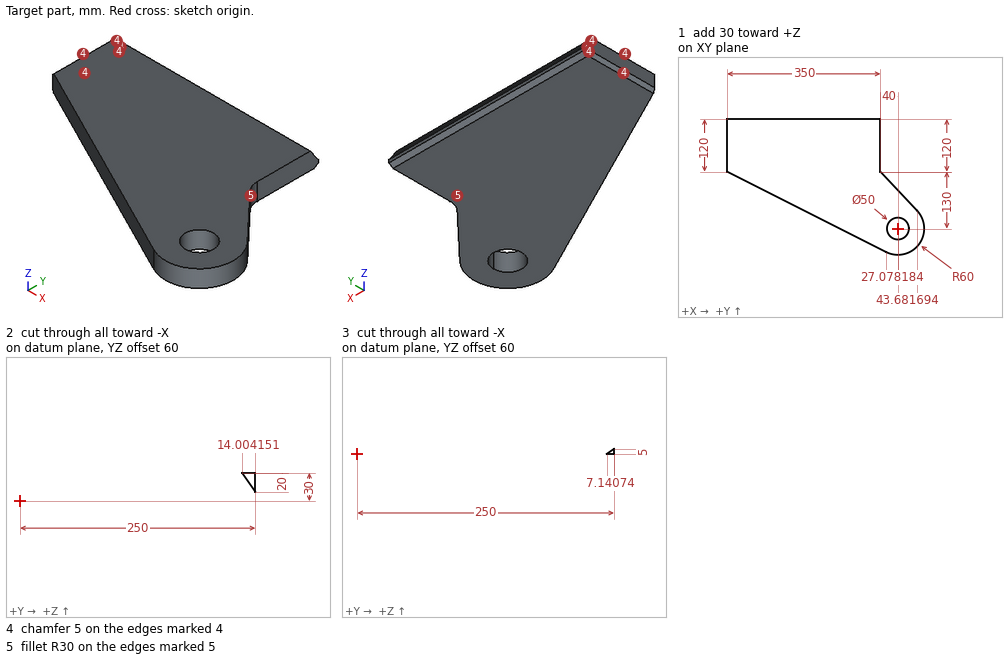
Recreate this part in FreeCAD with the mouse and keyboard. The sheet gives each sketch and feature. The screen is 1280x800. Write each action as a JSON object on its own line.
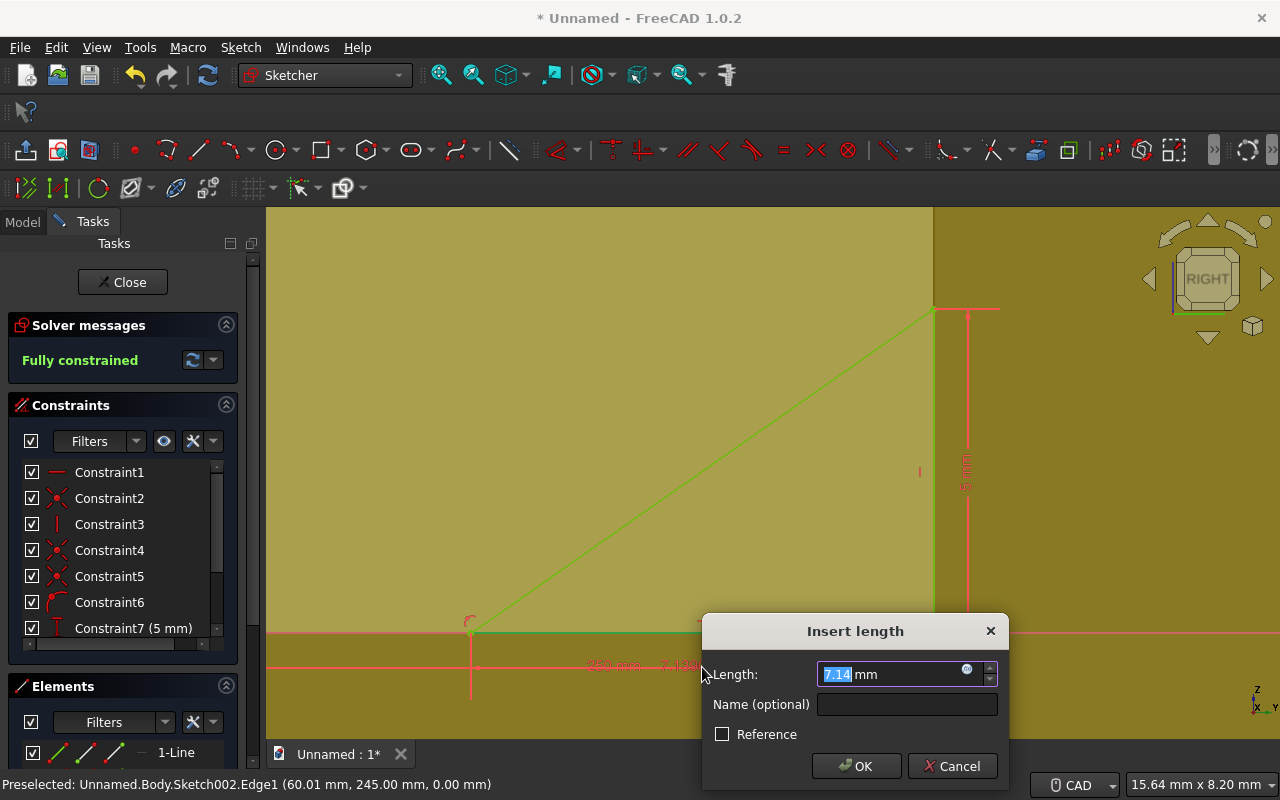
{"action": "type", "text": "7.14074"}
{"action": "key", "text": "Return"}
{"action": "key", "text": "Escape"}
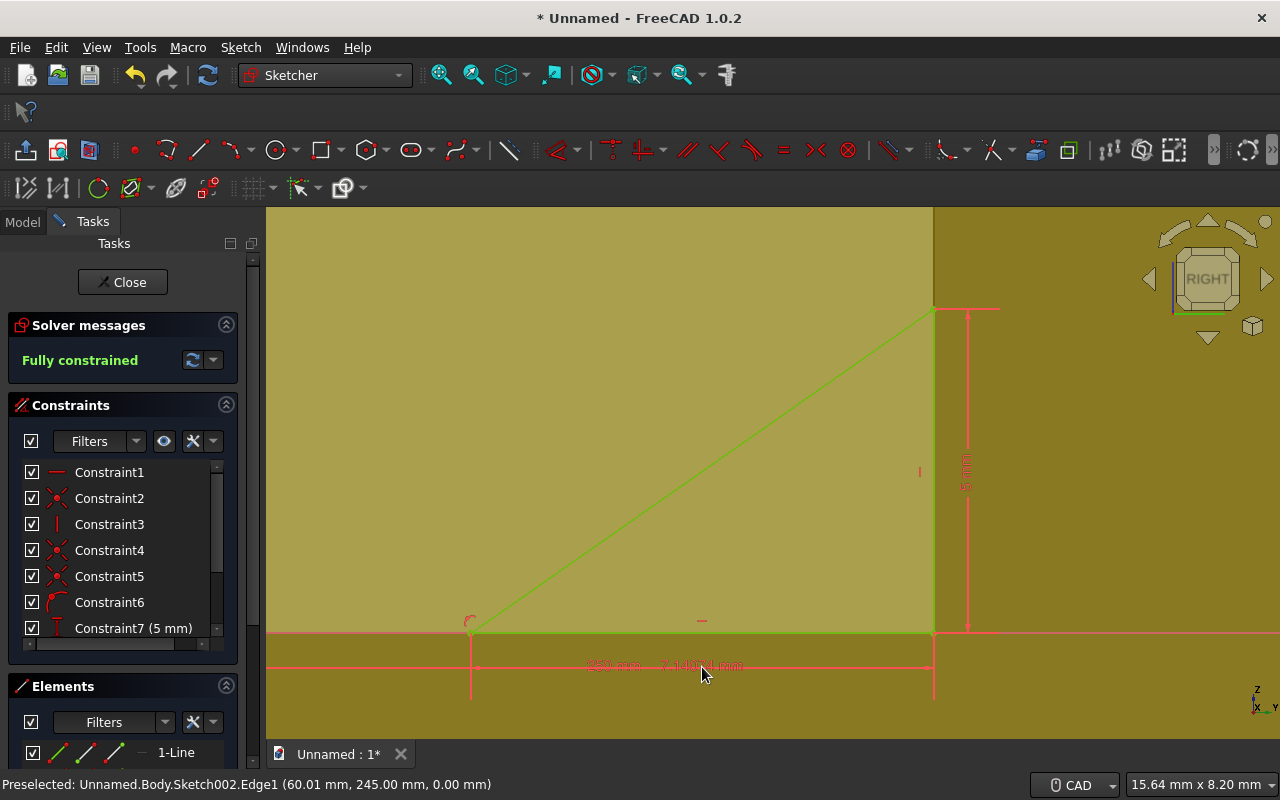
{"action": "left_click", "coordinate": [123, 282]}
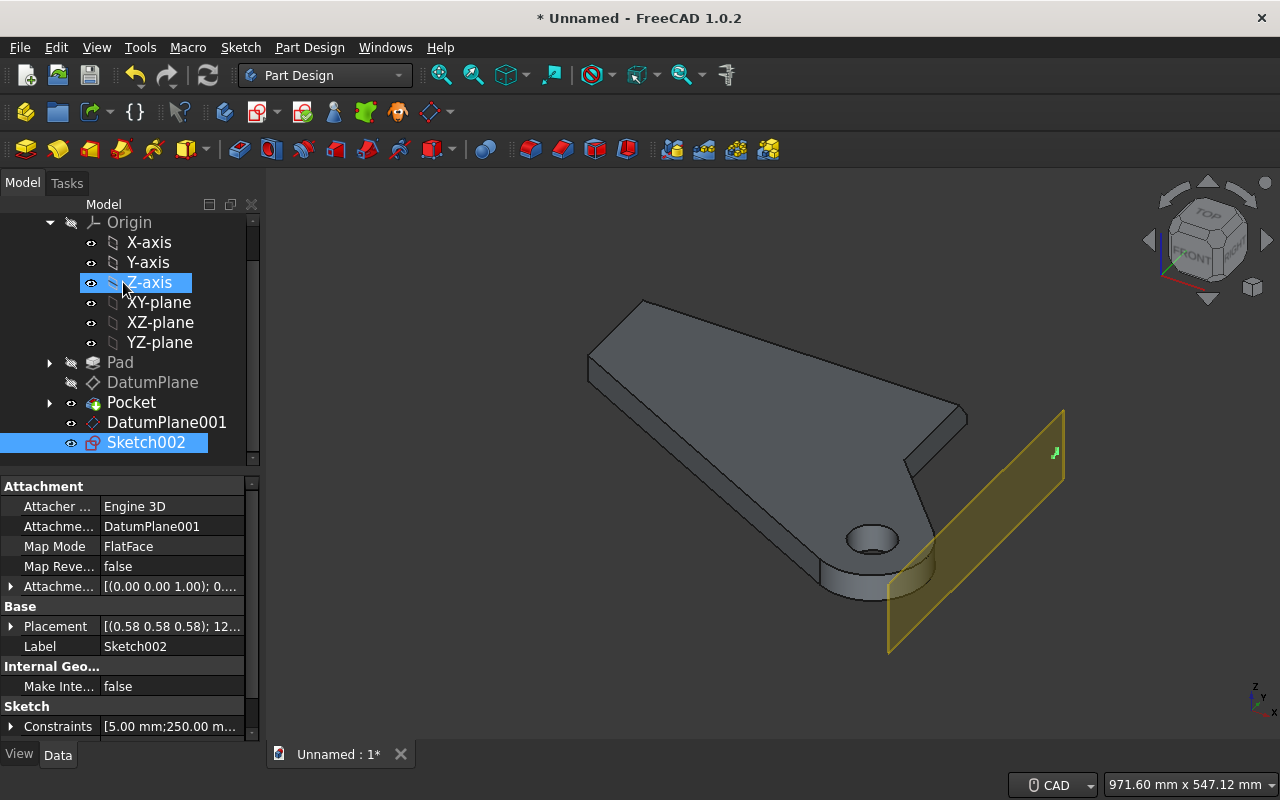
{"action": "left_click", "coordinate": [240, 150]}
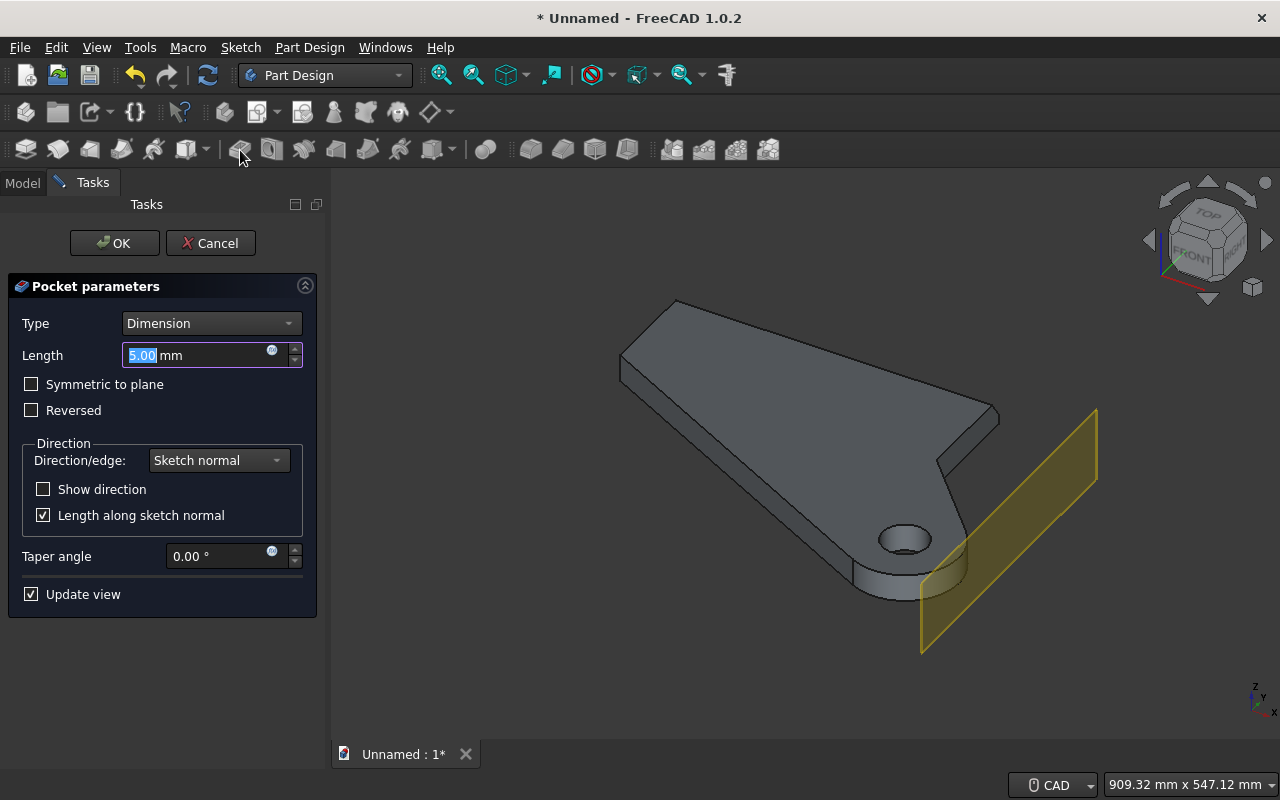
{"action": "left_click", "coordinate": [212, 324]}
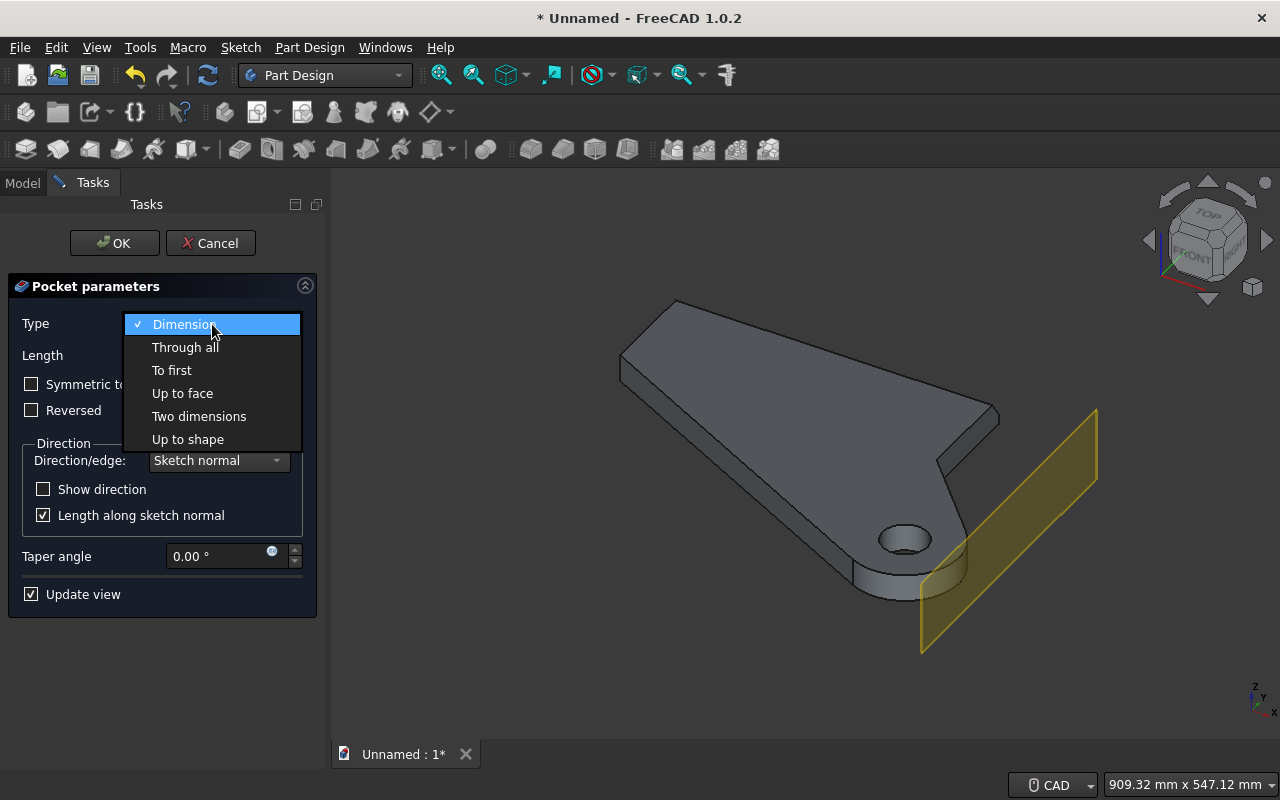
{"action": "left_click", "coordinate": [212, 348]}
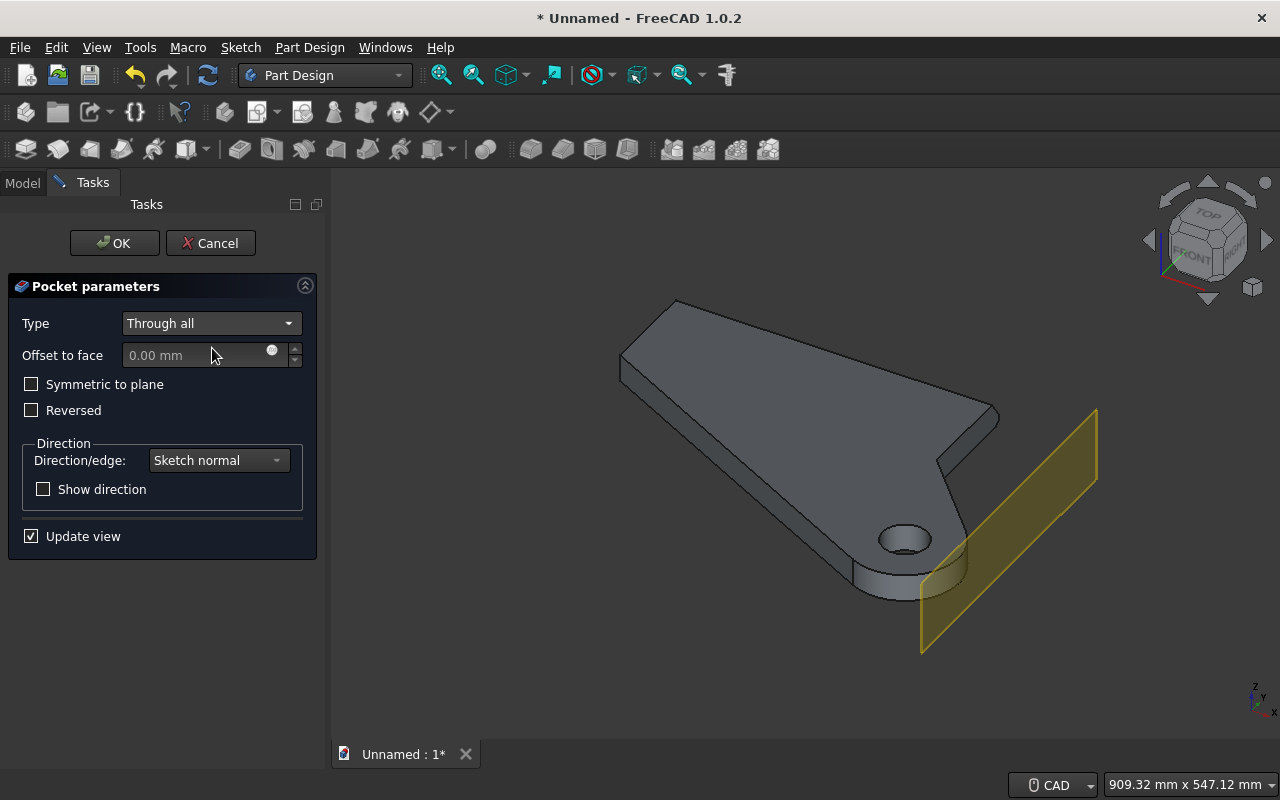
{"action": "left_click", "coordinate": [115, 243]}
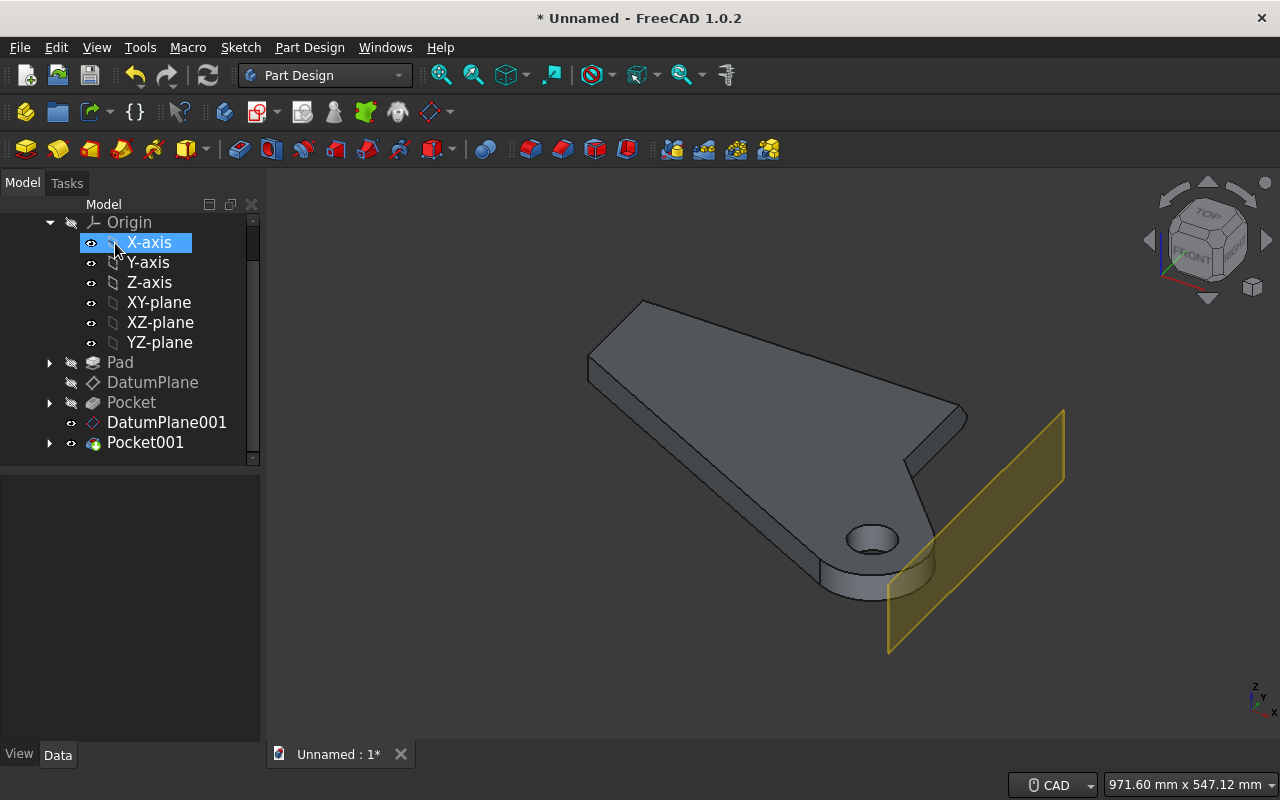
{"action": "left_click", "coordinate": [116, 423]}
{"action": "key", "text": "space"}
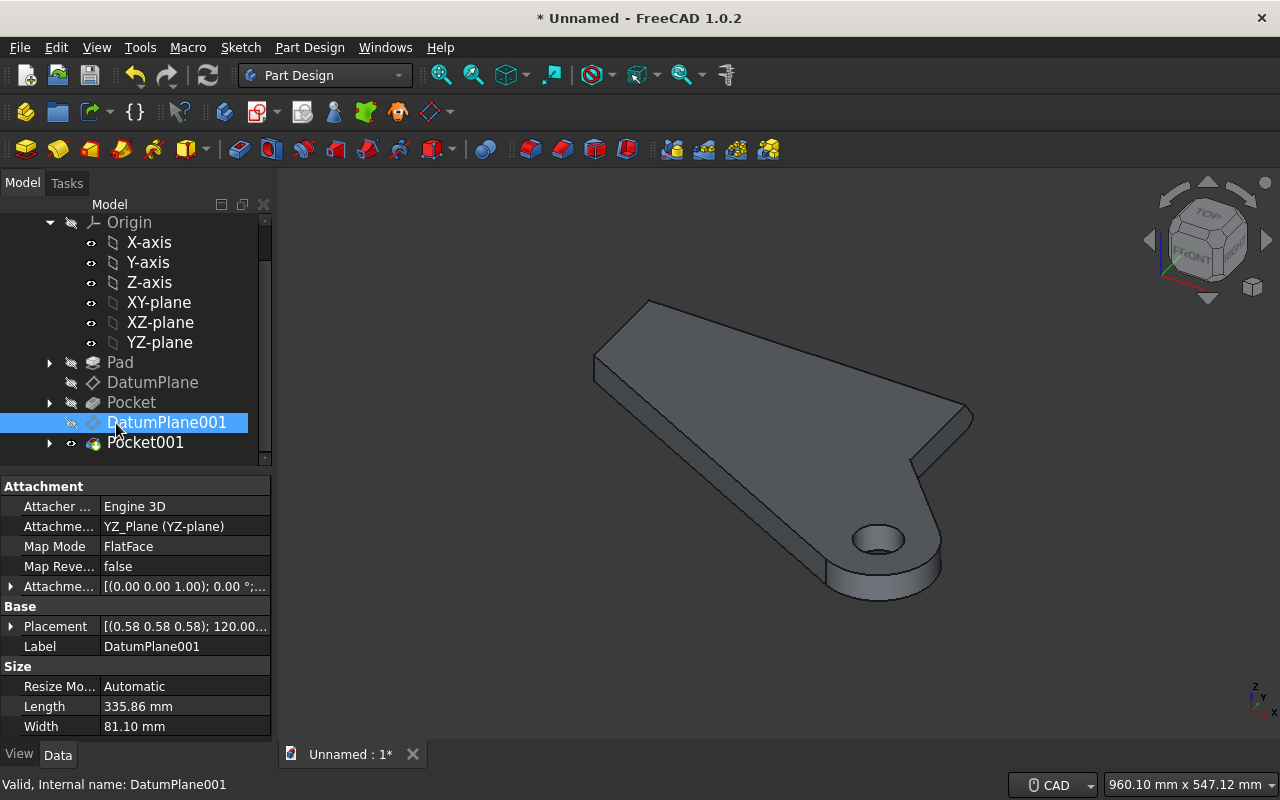
{"action": "key", "text": "0"}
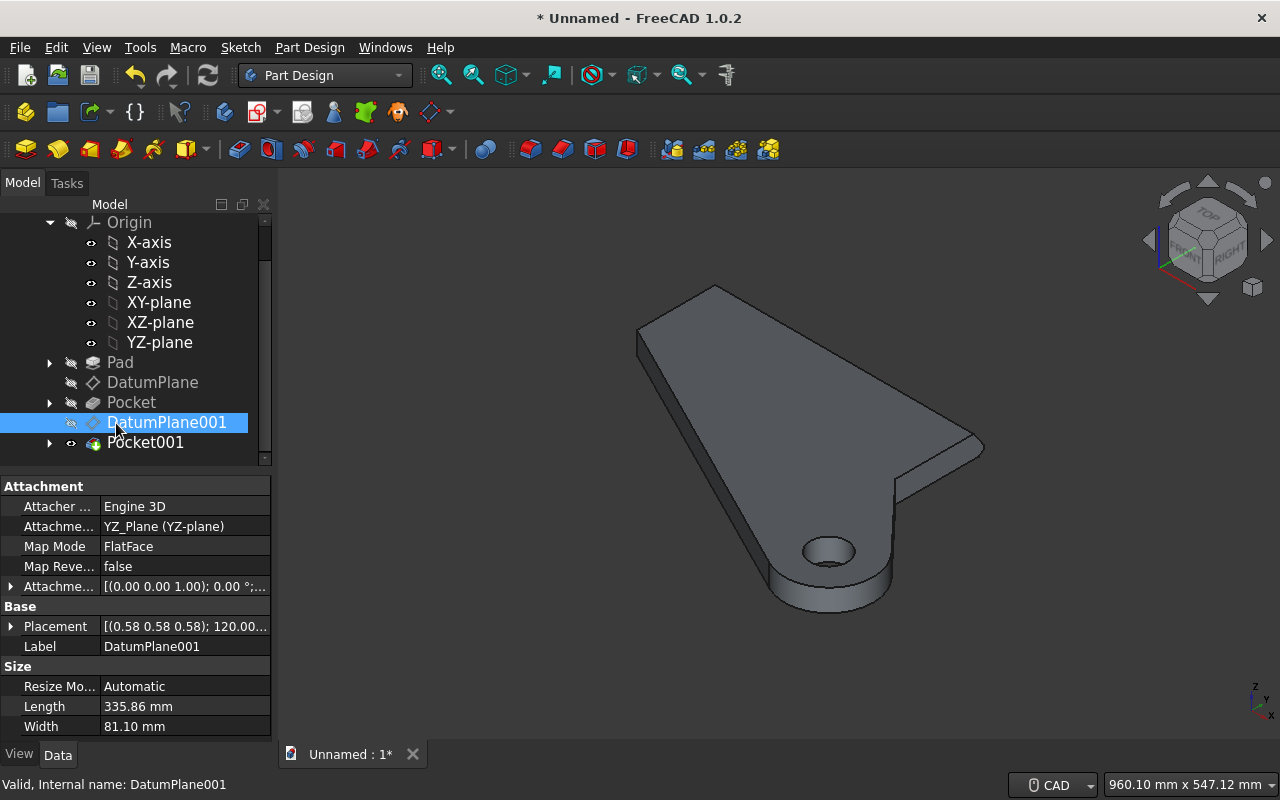
{"action": "key", "text": "2"}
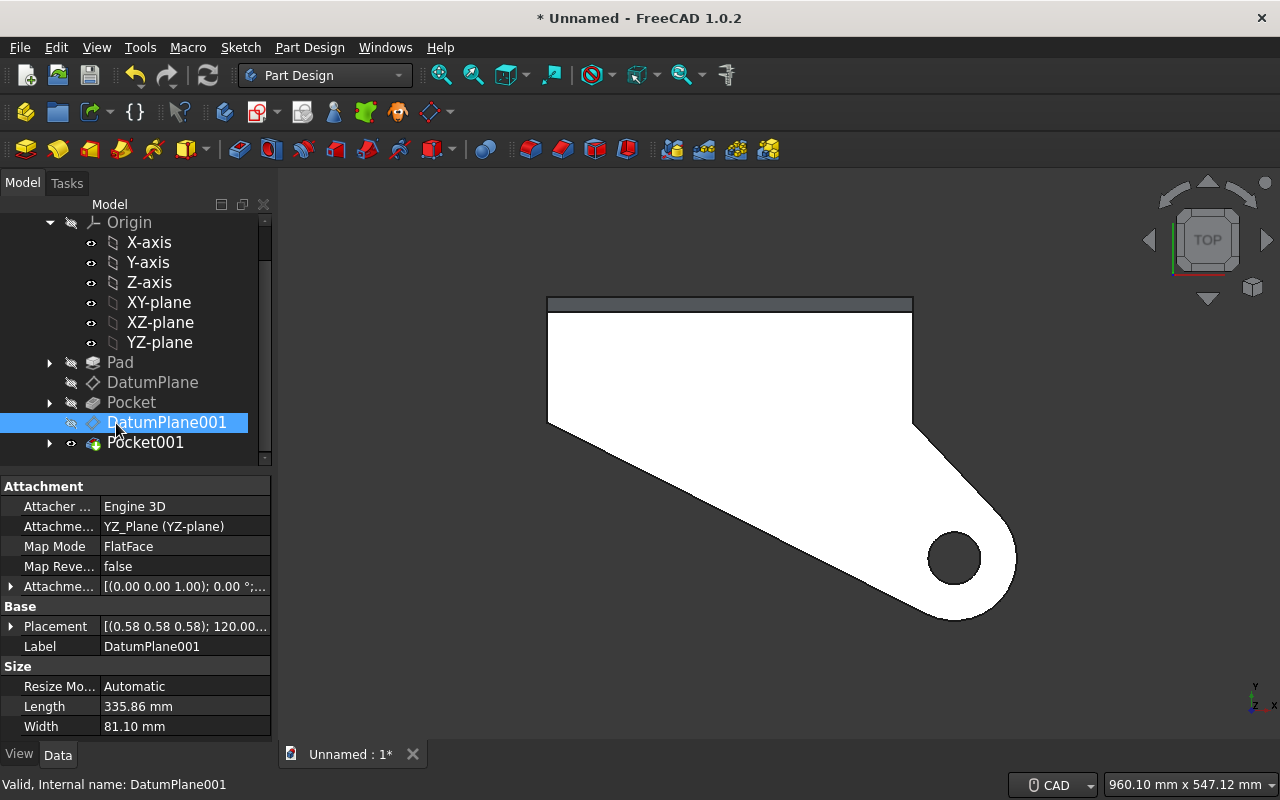
{"action": "left_click", "coordinate": [547, 366]}